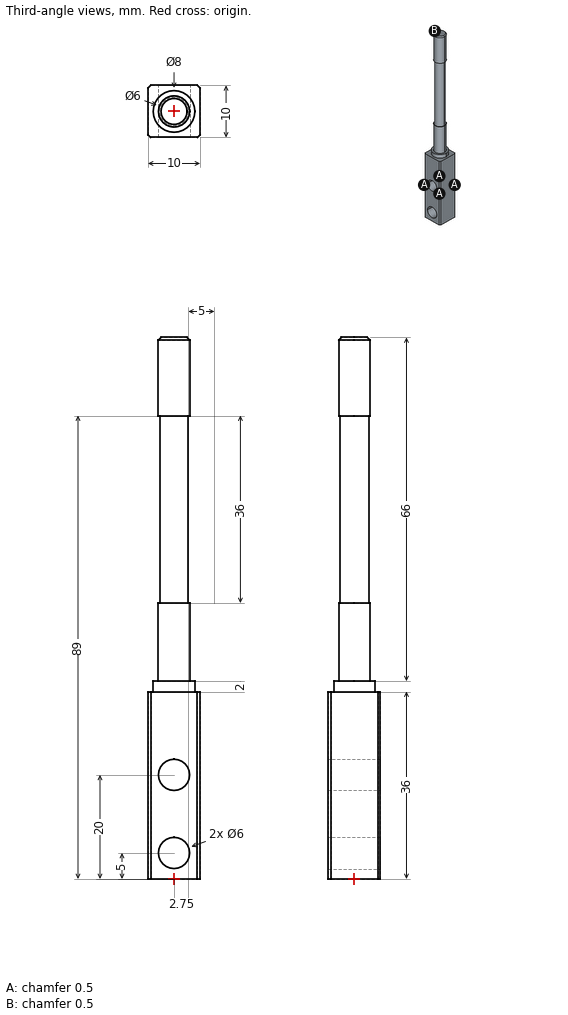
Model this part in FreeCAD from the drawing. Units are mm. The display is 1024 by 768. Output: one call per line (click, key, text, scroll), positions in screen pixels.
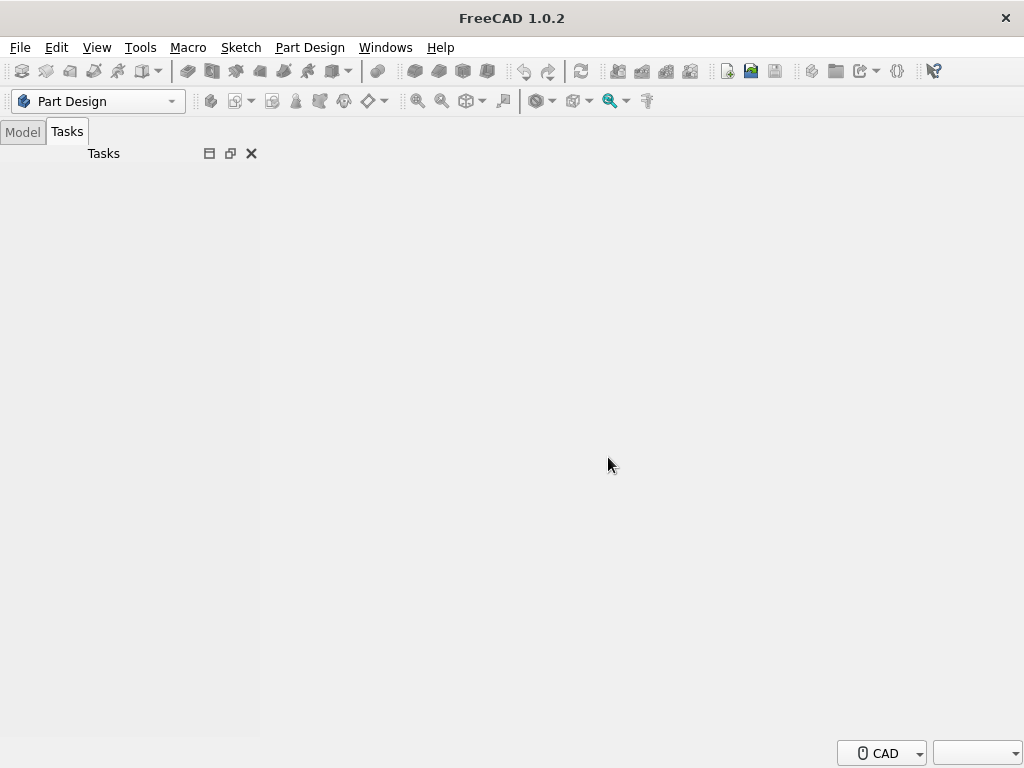
key(ctrl+n)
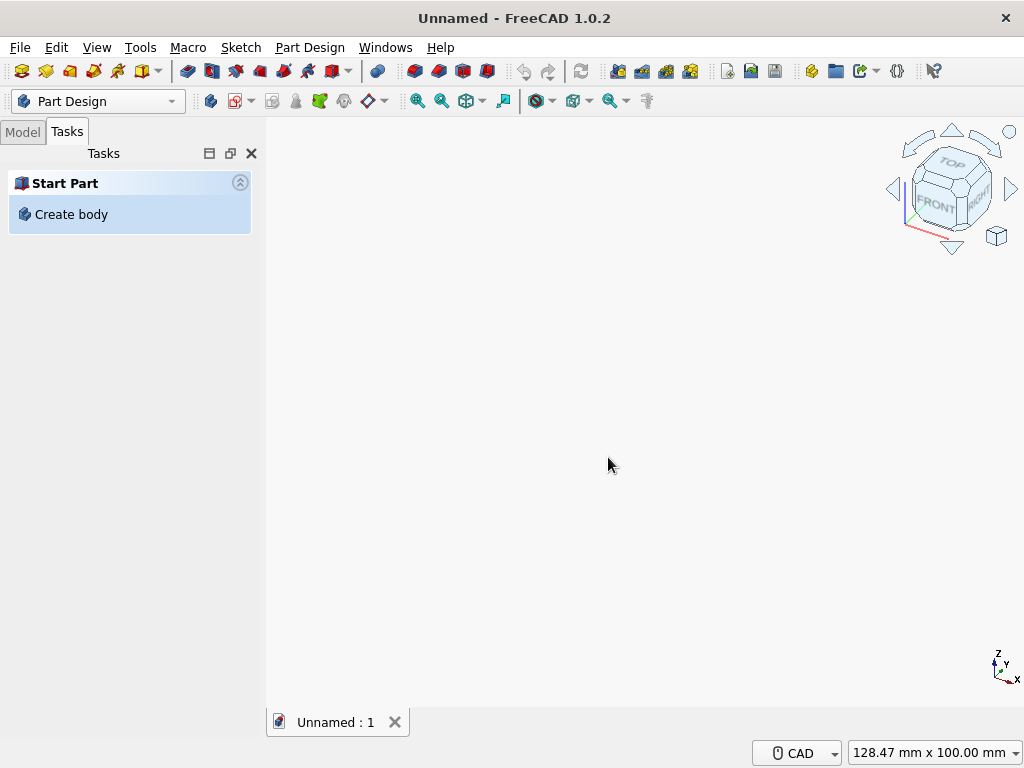
click(236, 102)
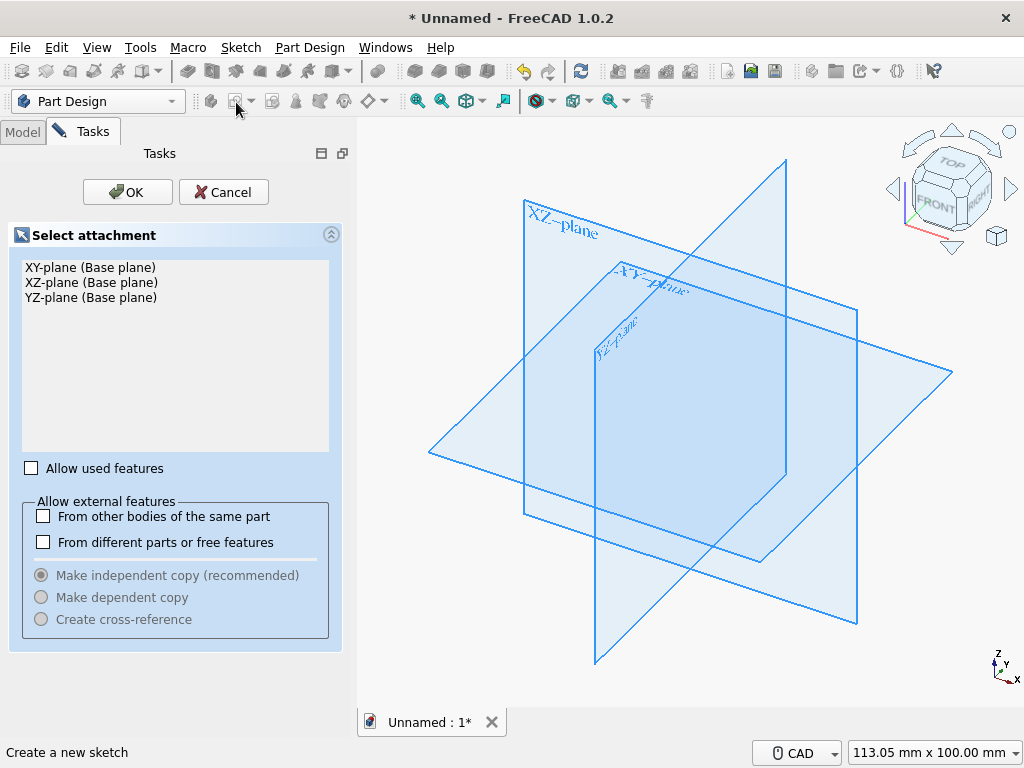
click(82, 268)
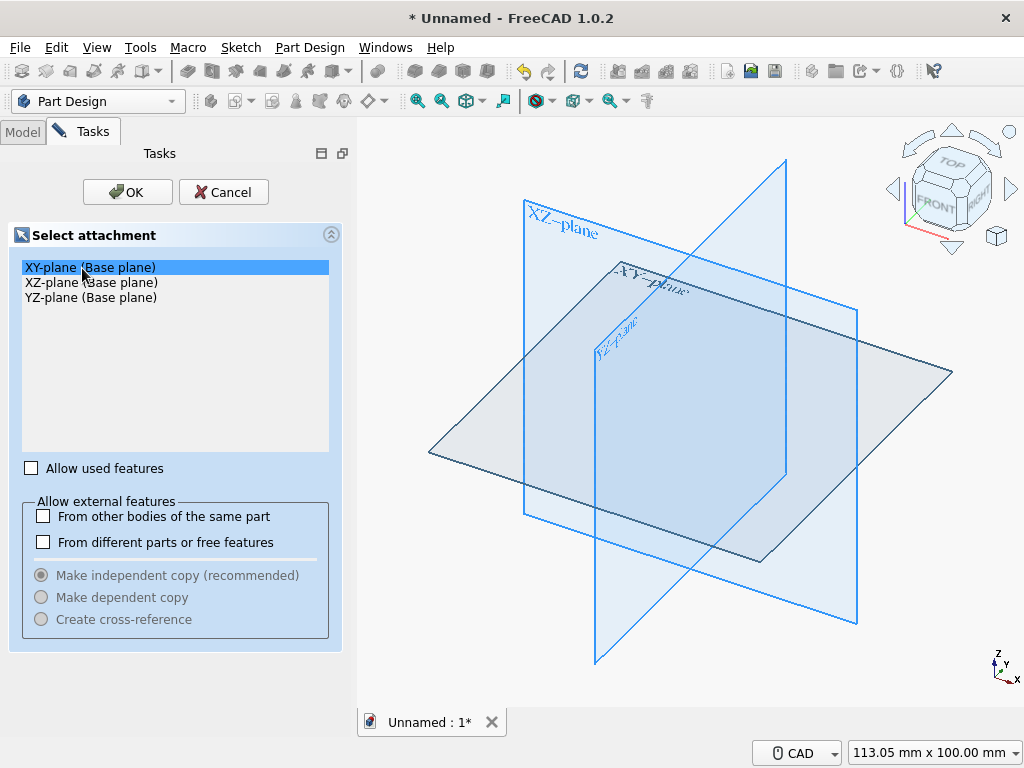
click(128, 192)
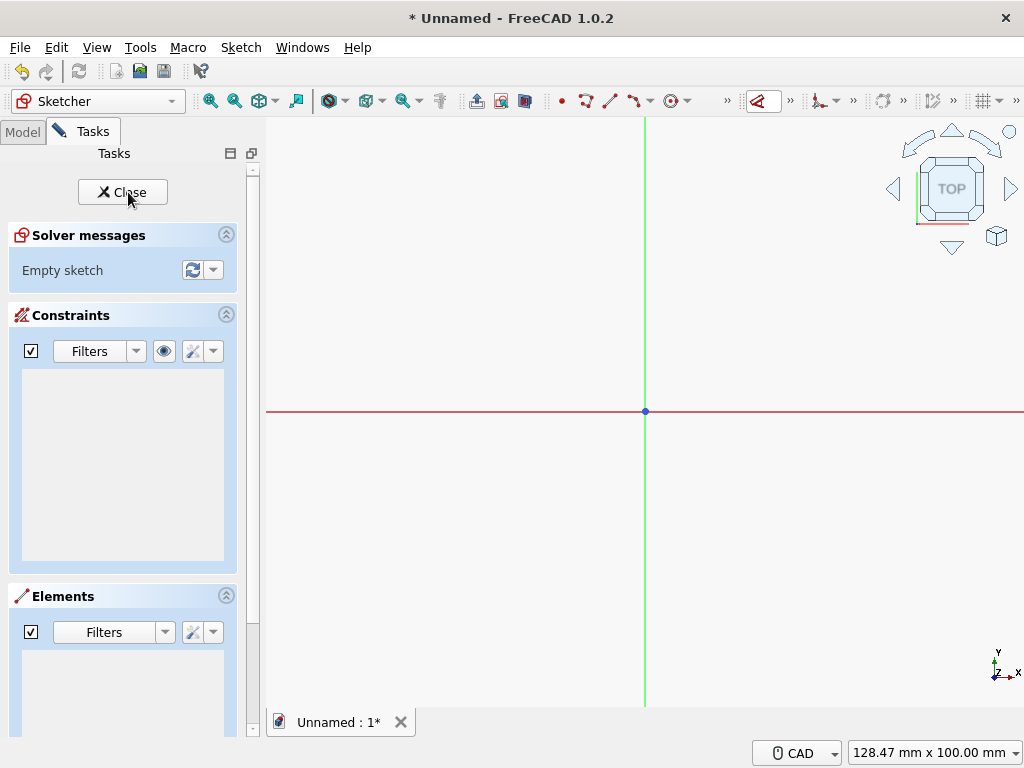
scroll(659, 412, up, 9)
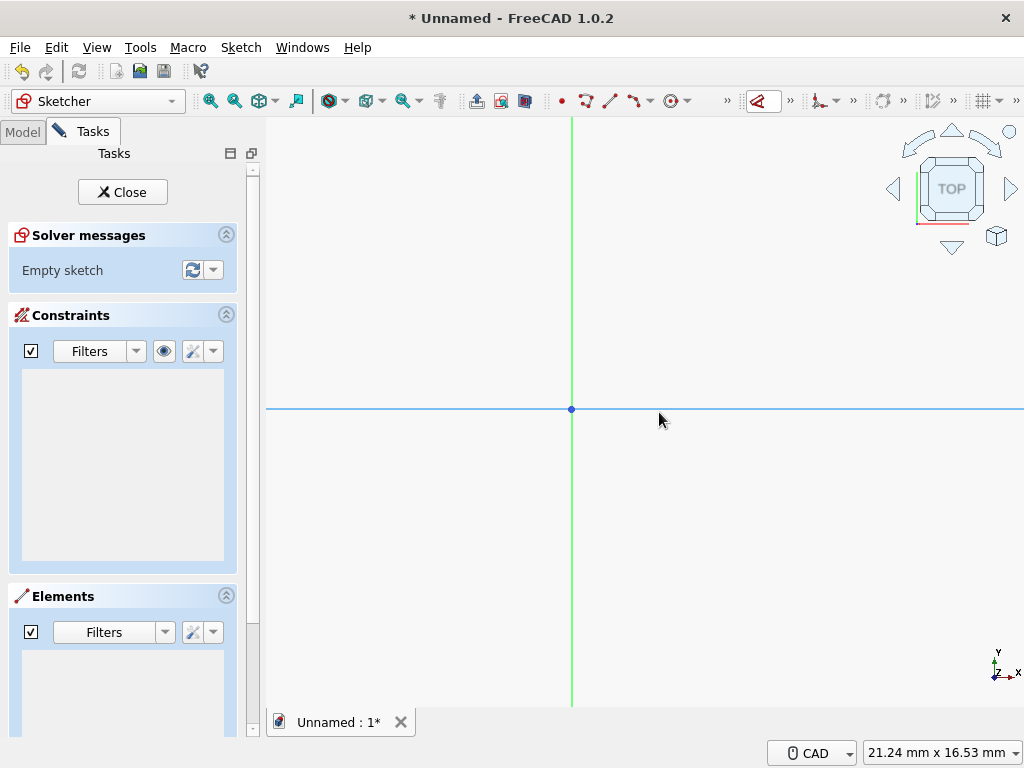
key(g)
key(v)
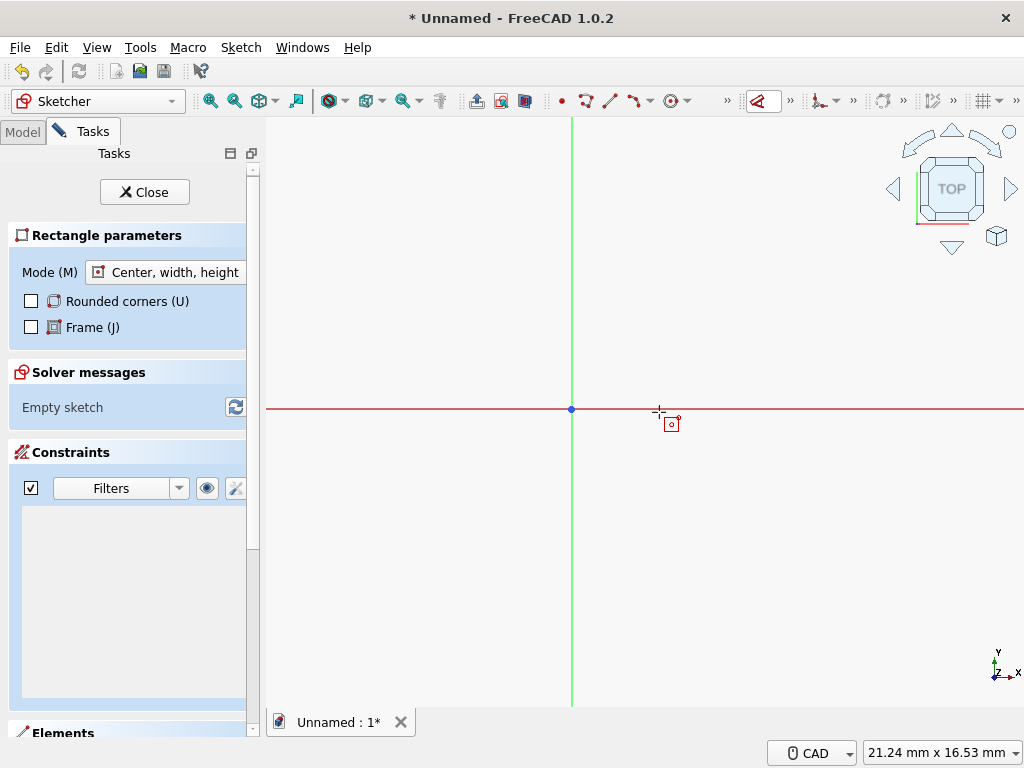
click(572, 409)
click(750, 231)
key(Escape)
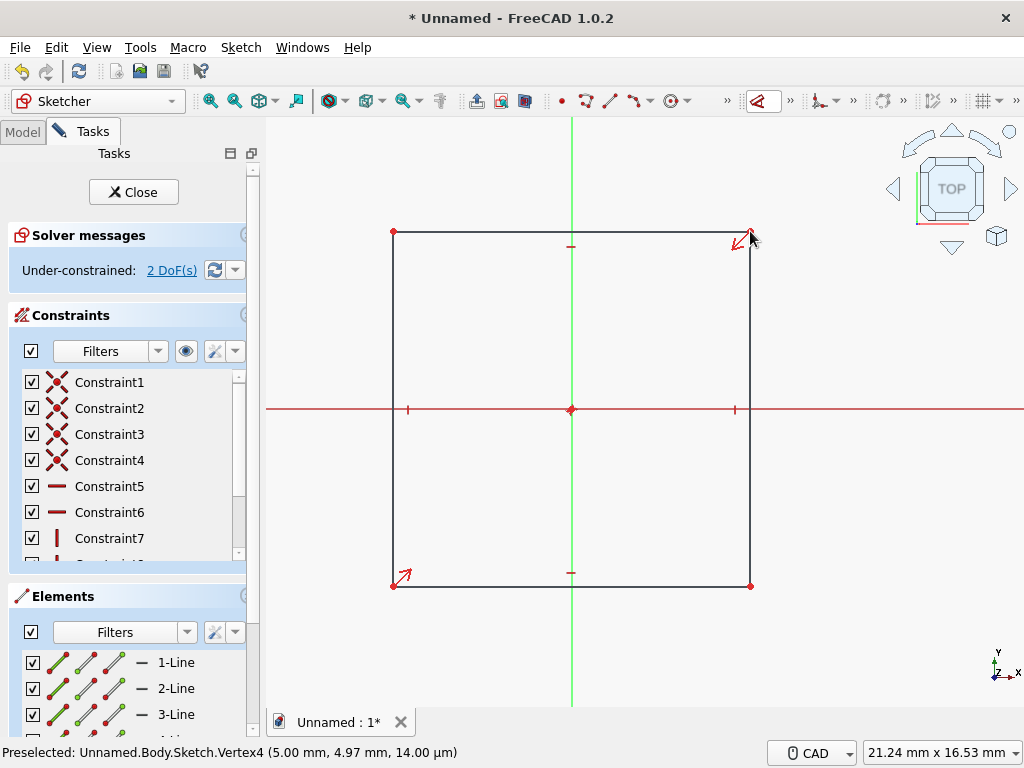
key(d)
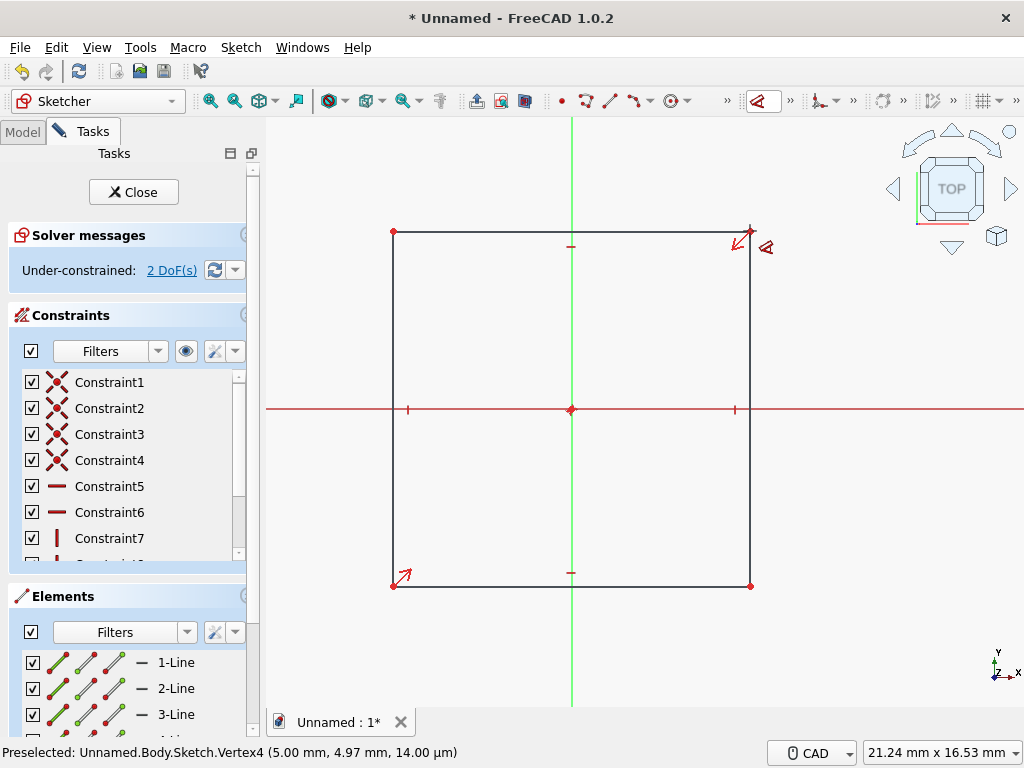
click(500, 587)
click(490, 621)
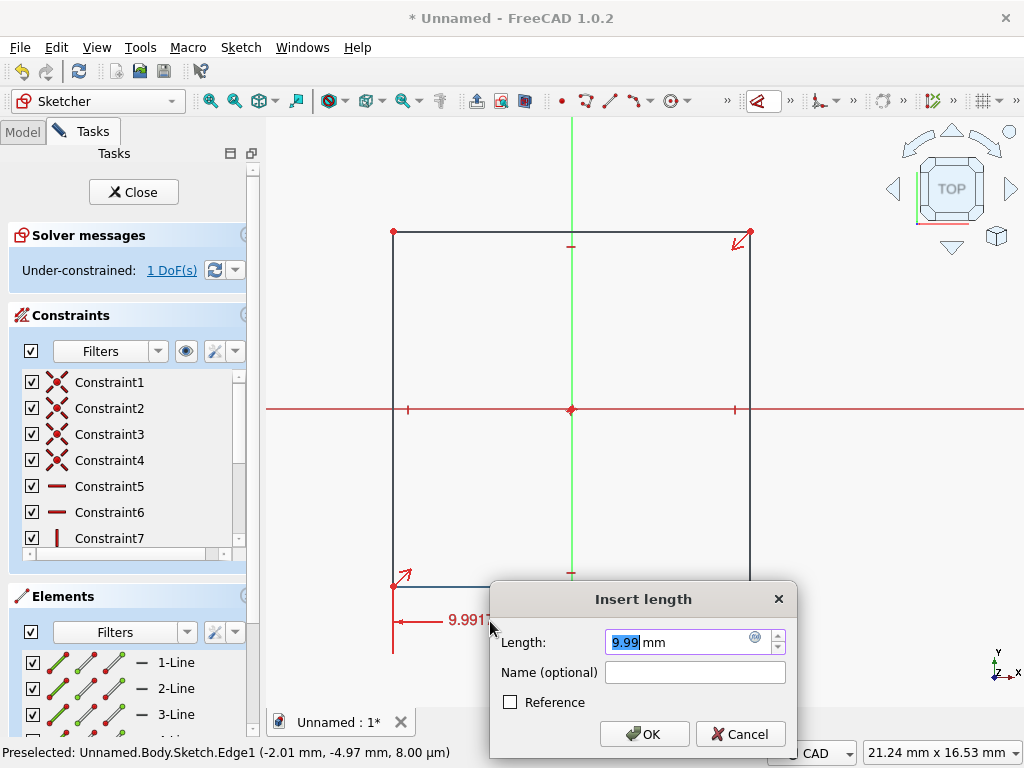
text(10)
key(Return)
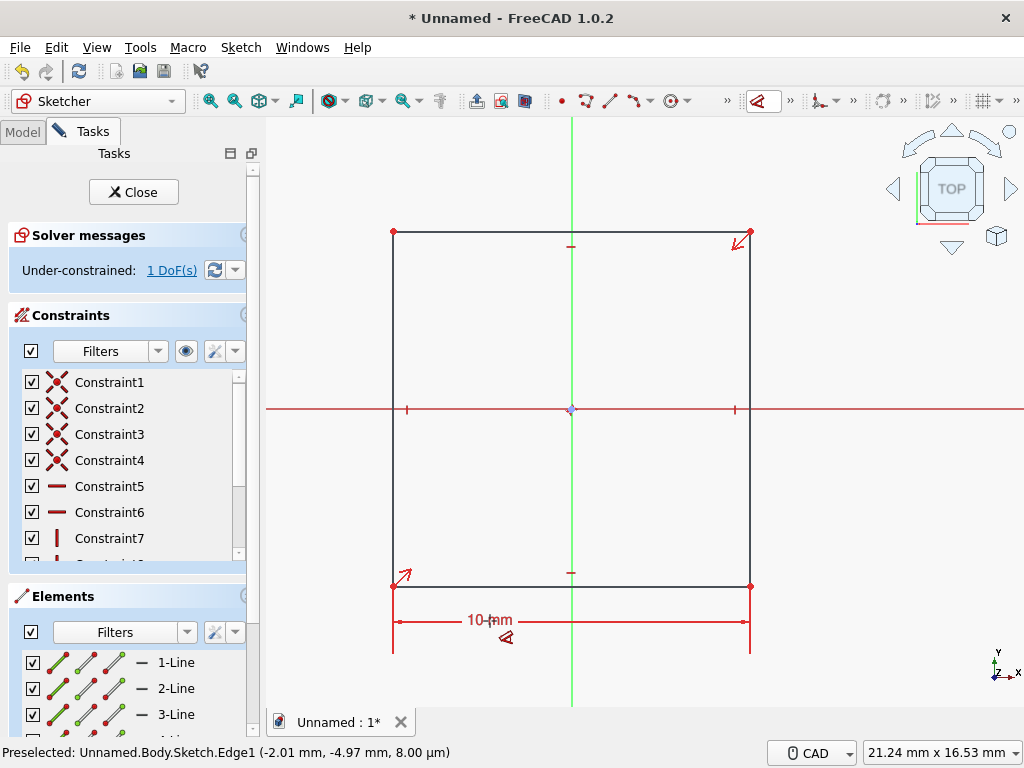
click(750, 480)
click(784, 328)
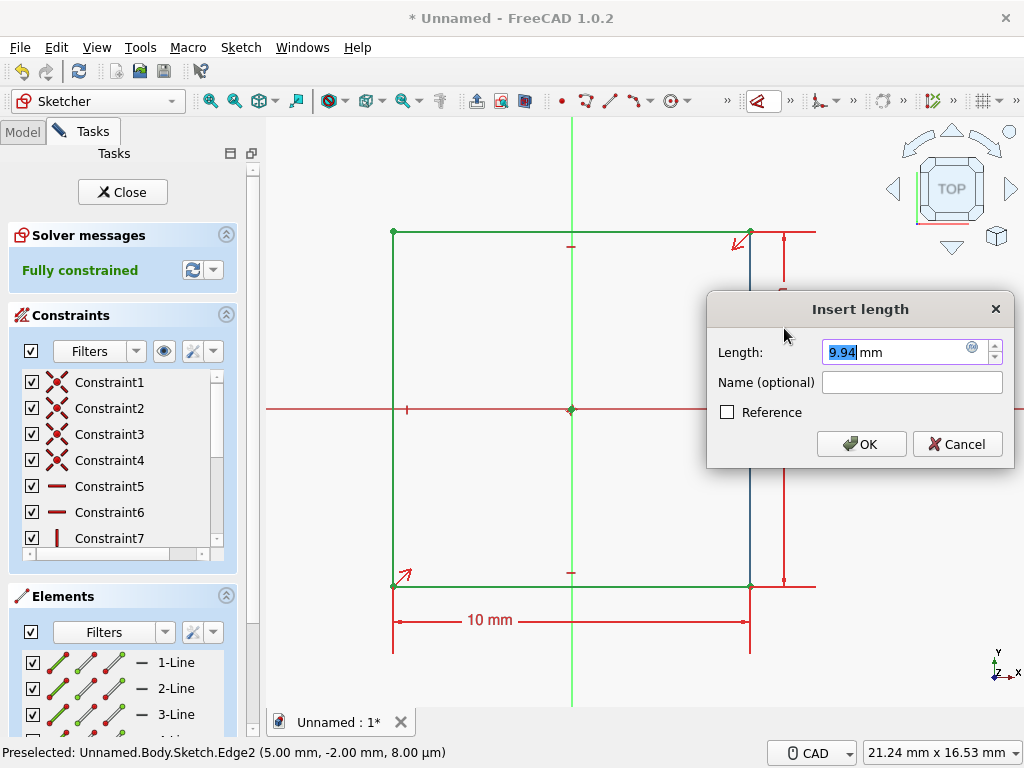
text(10)
key(Return)
key(Escape)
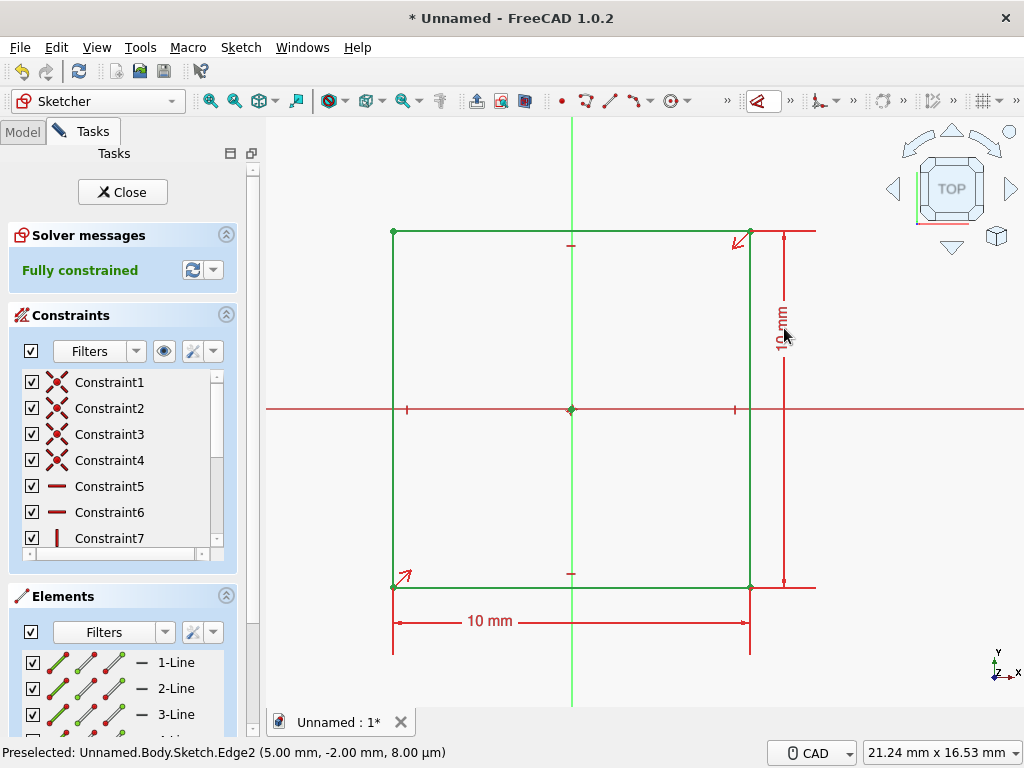
click(123, 192)